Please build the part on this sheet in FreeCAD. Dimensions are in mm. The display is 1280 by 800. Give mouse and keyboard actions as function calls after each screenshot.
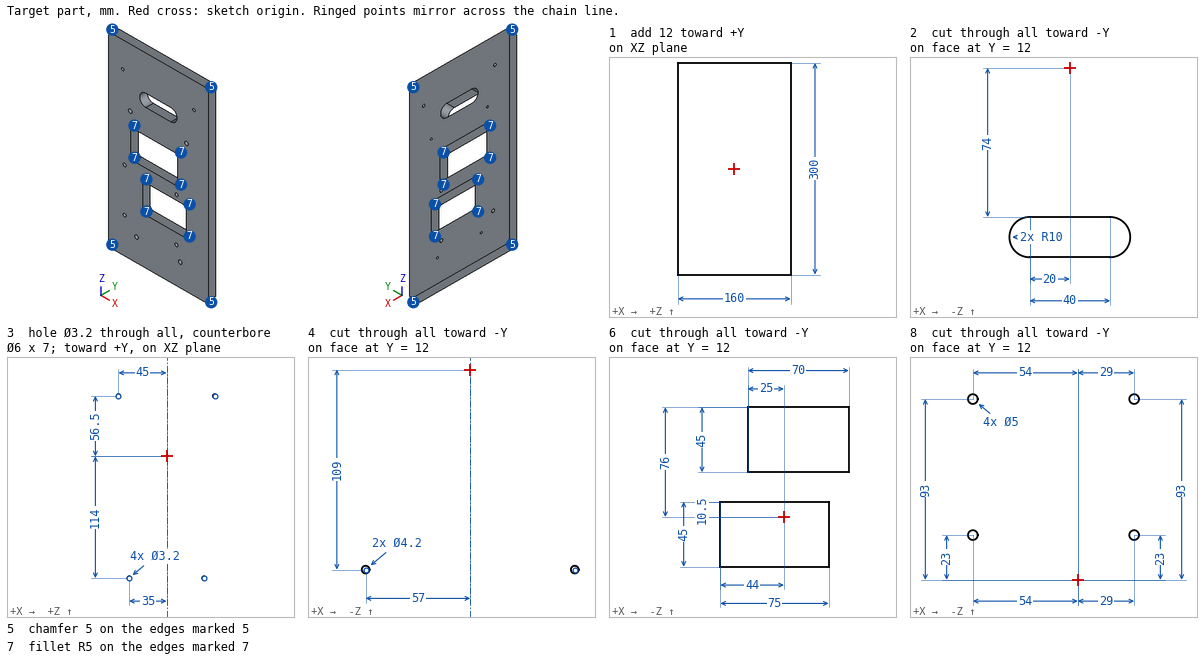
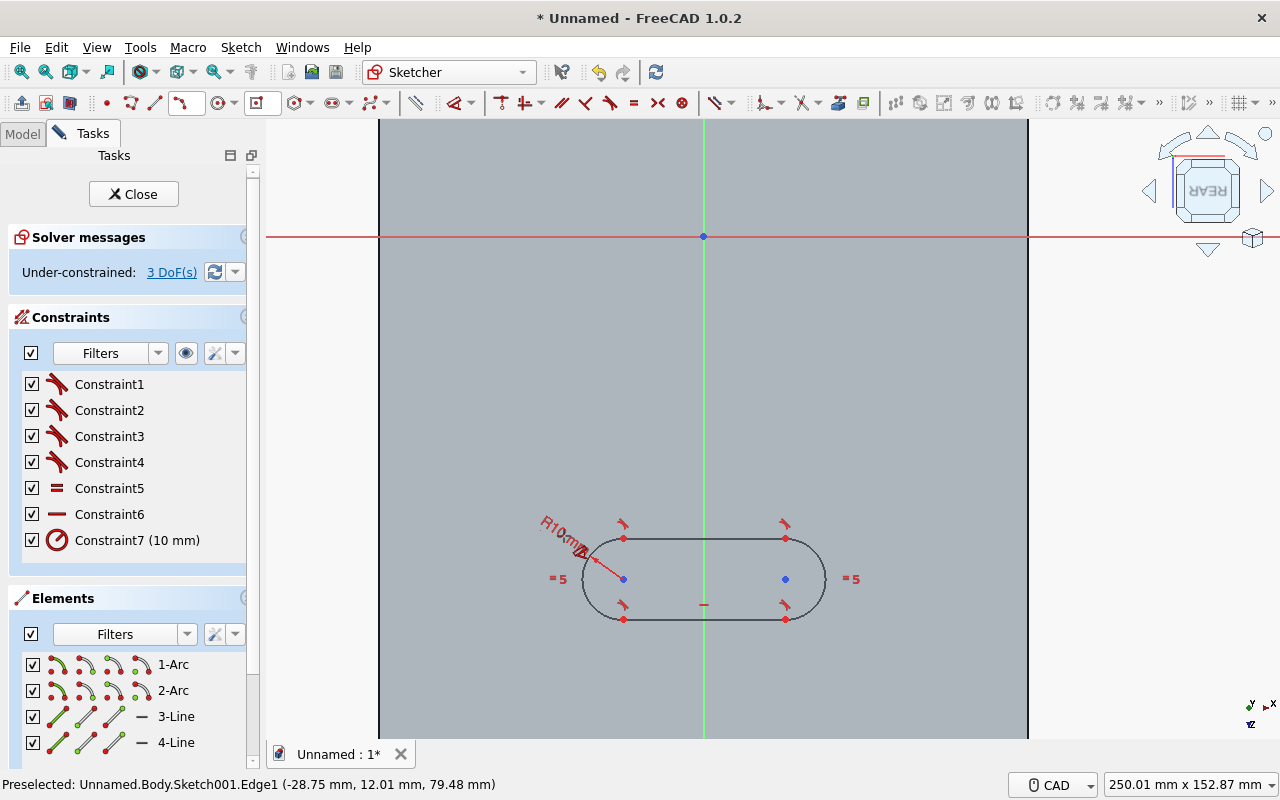
click(672, 539)
click(667, 573)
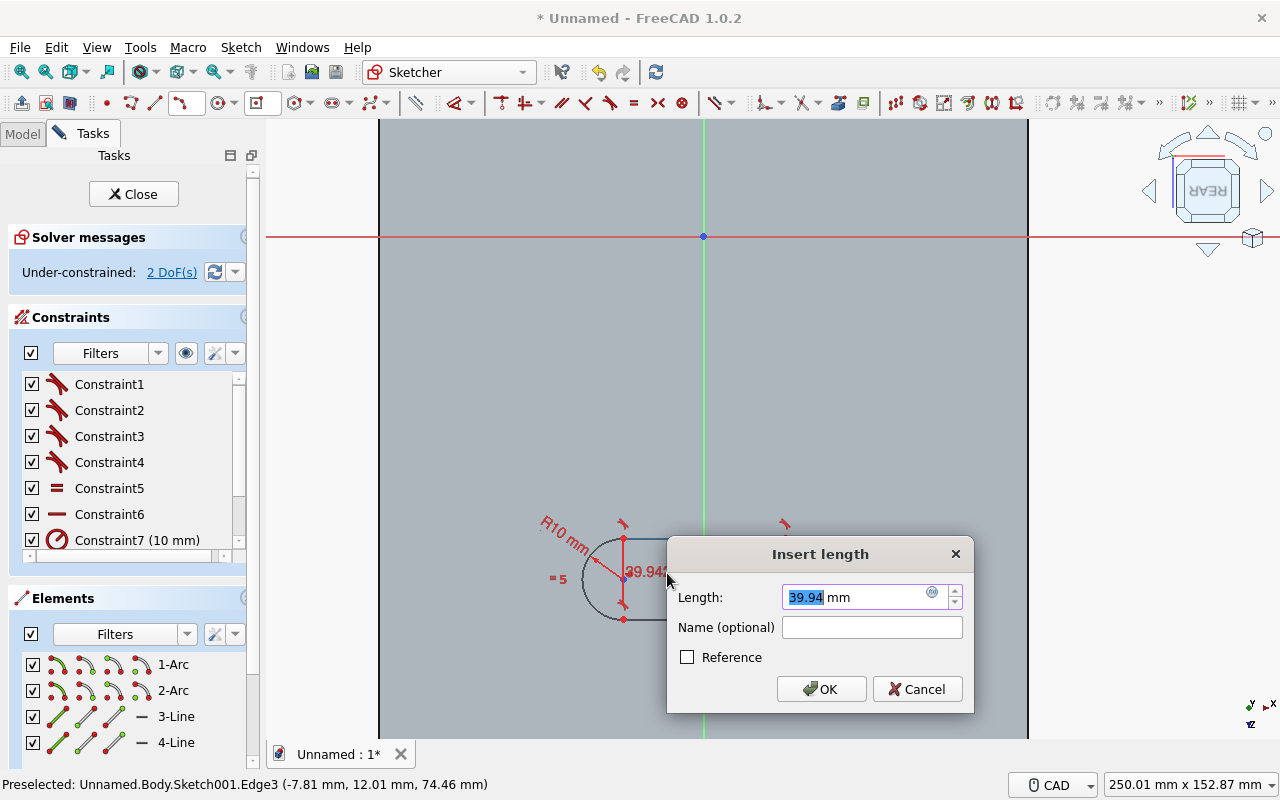
text(40)
key(Return)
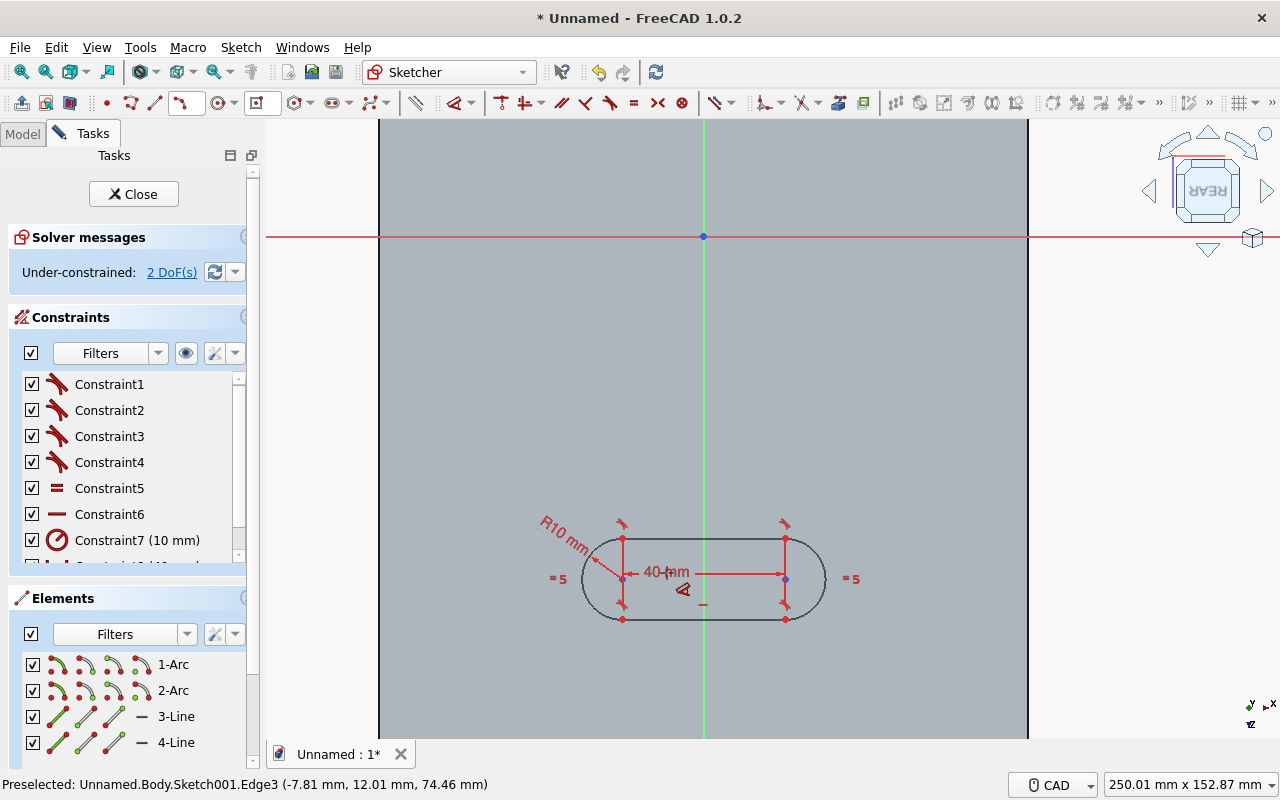
click(623, 539)
click(663, 203)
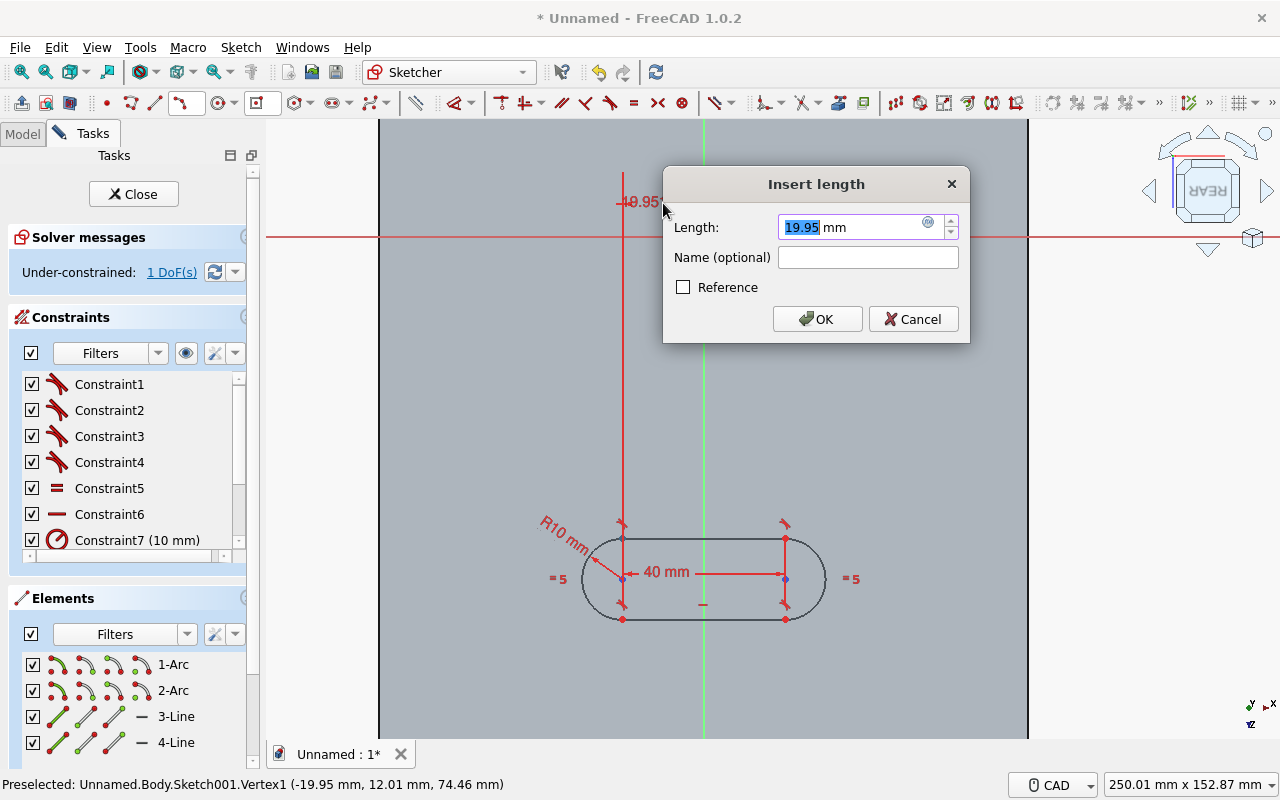
text(20)
key(Return)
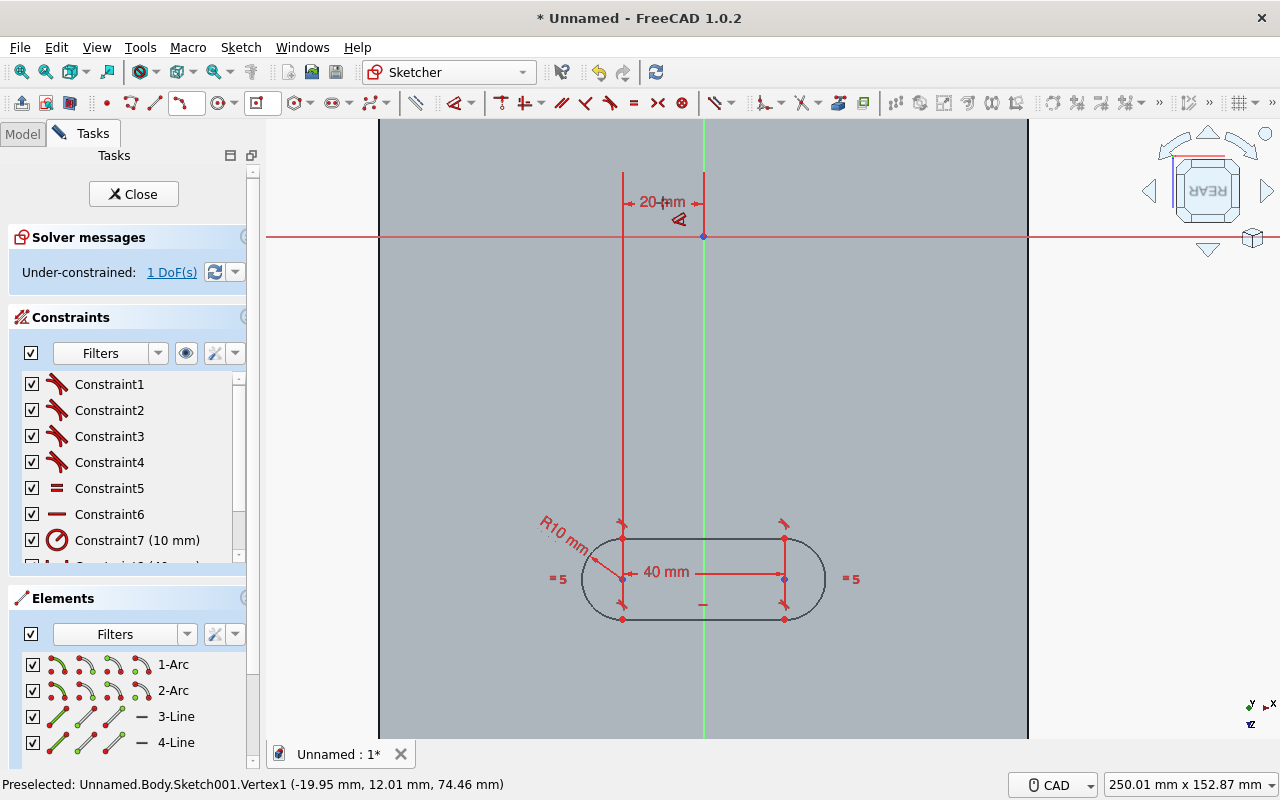
click(623, 539)
click(589, 388)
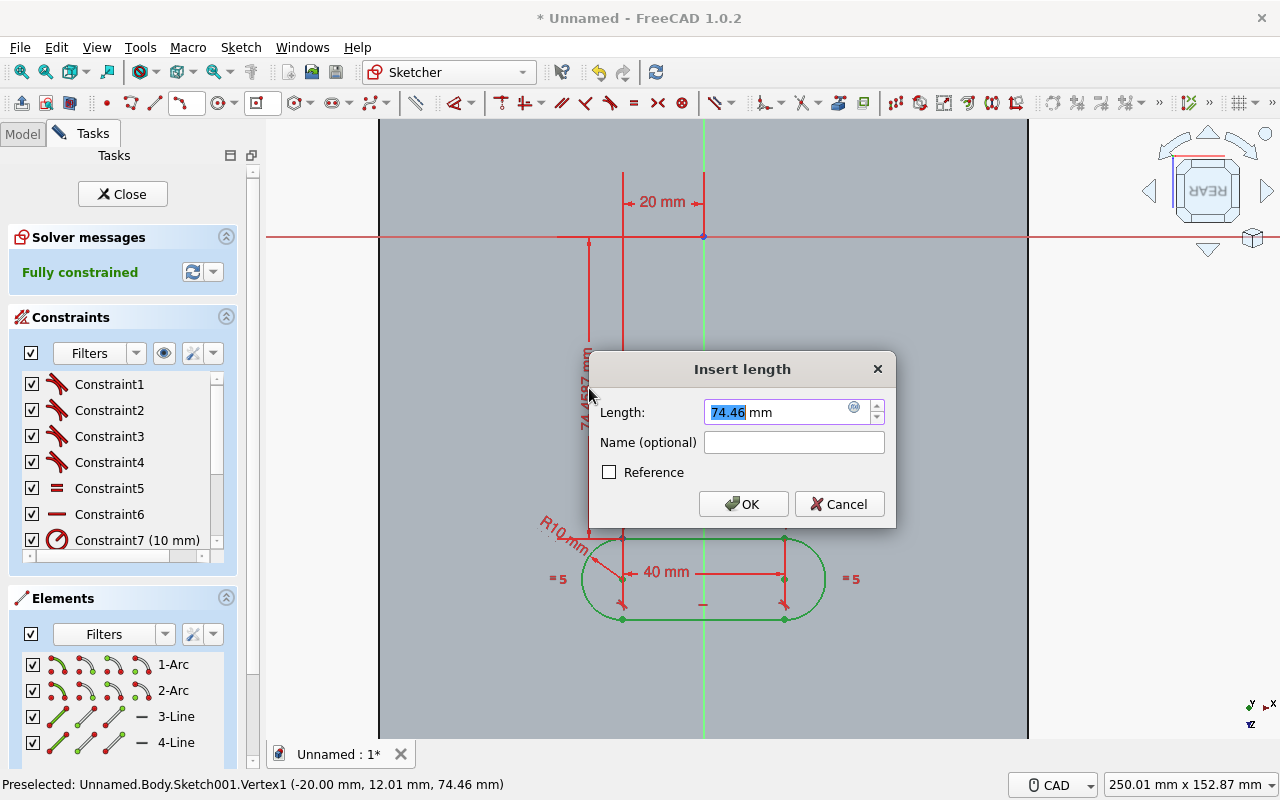
text(74)
key(Return)
key(Escape)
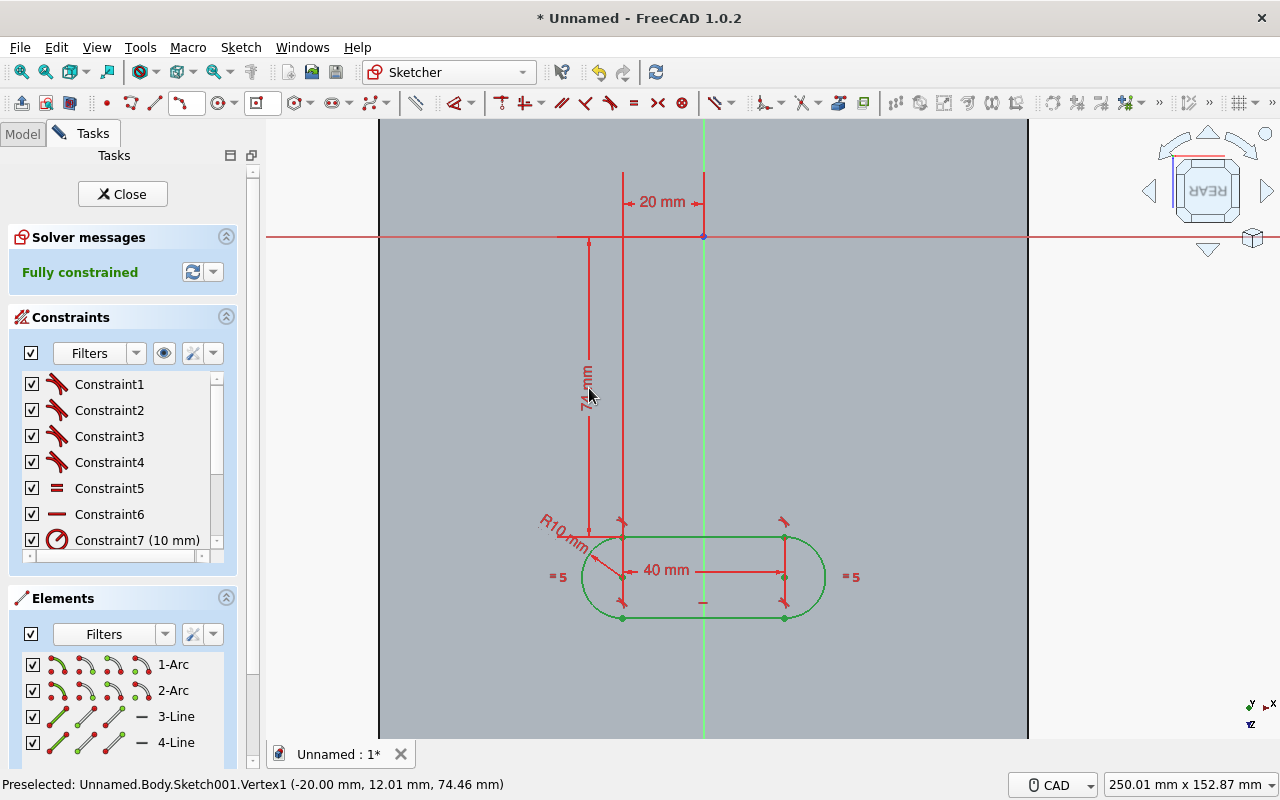
click(123, 194)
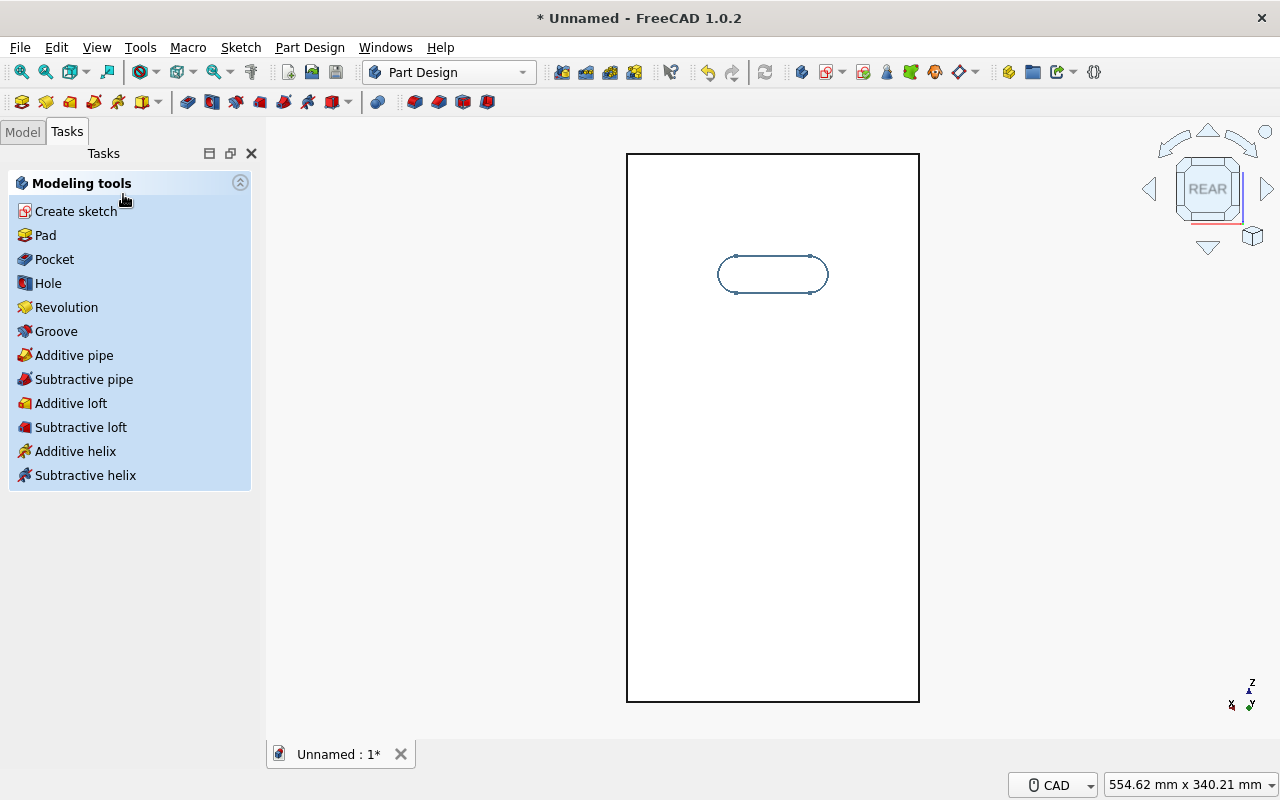
click(188, 102)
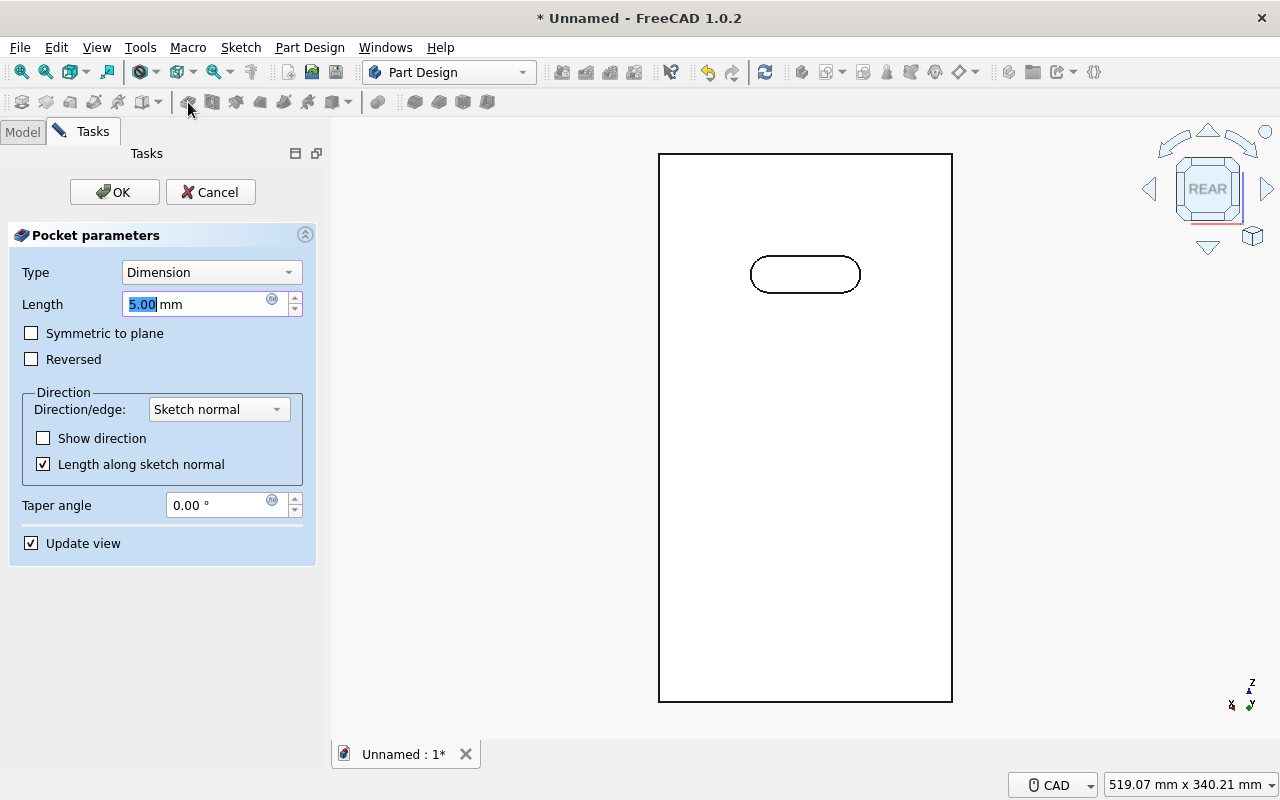
click(212, 272)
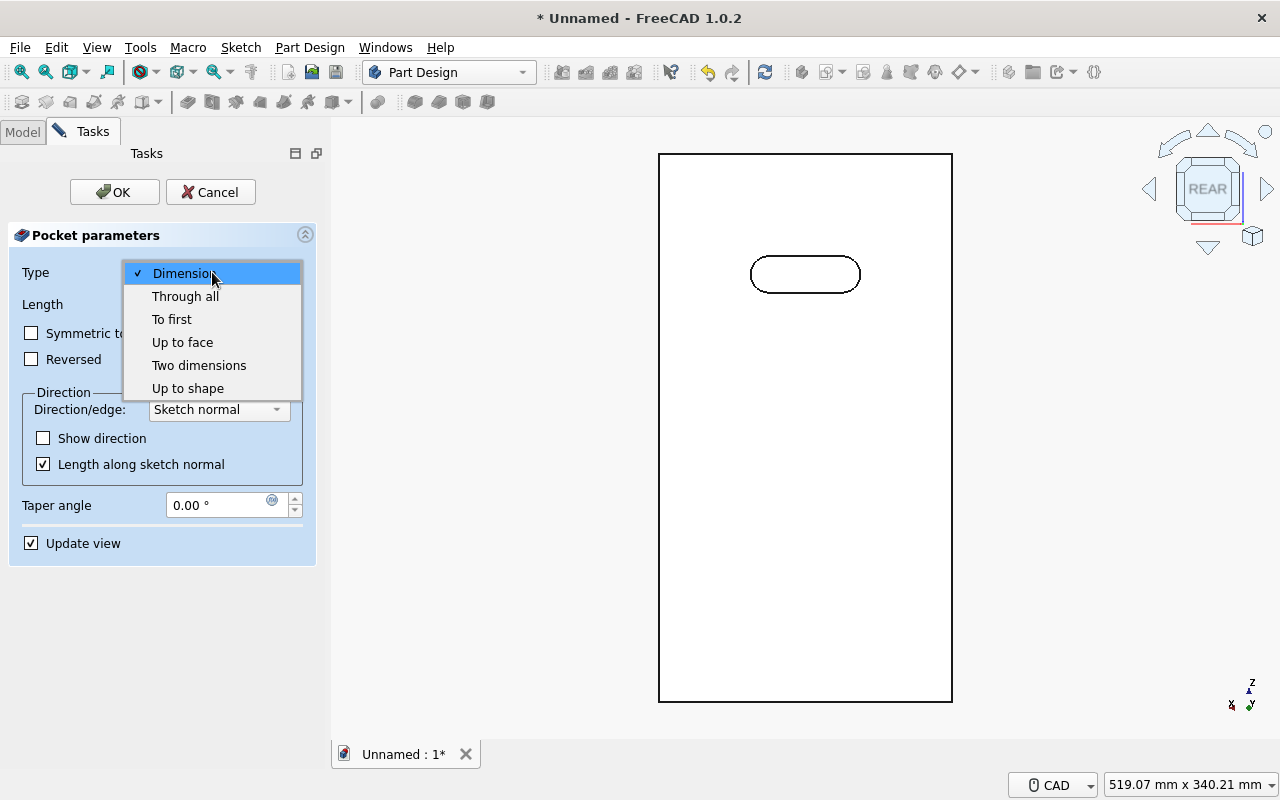
click(212, 296)